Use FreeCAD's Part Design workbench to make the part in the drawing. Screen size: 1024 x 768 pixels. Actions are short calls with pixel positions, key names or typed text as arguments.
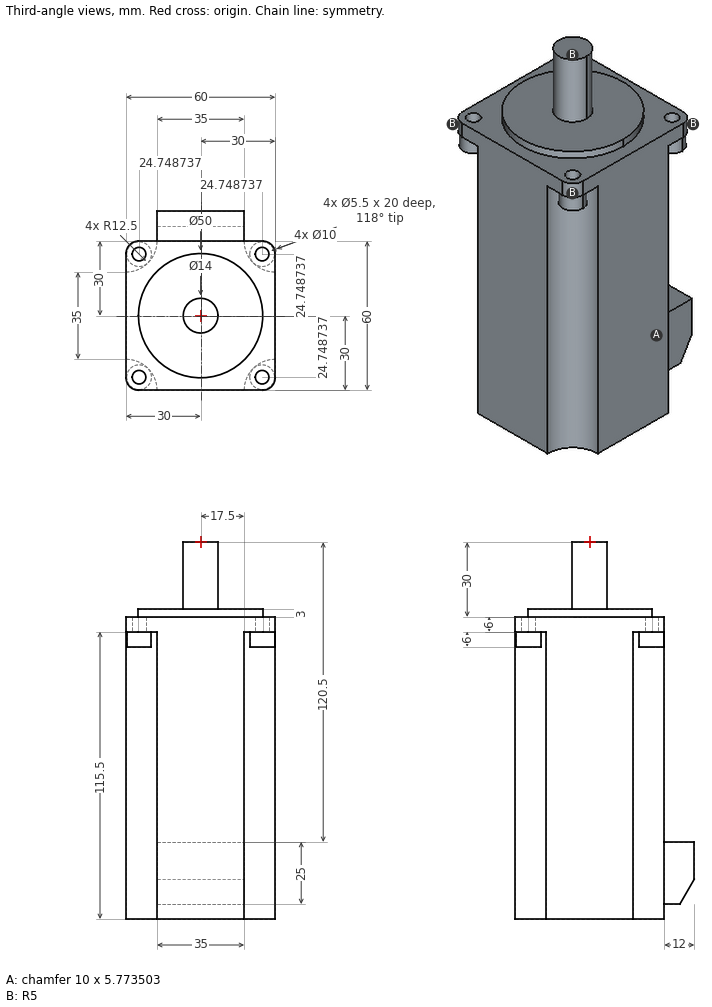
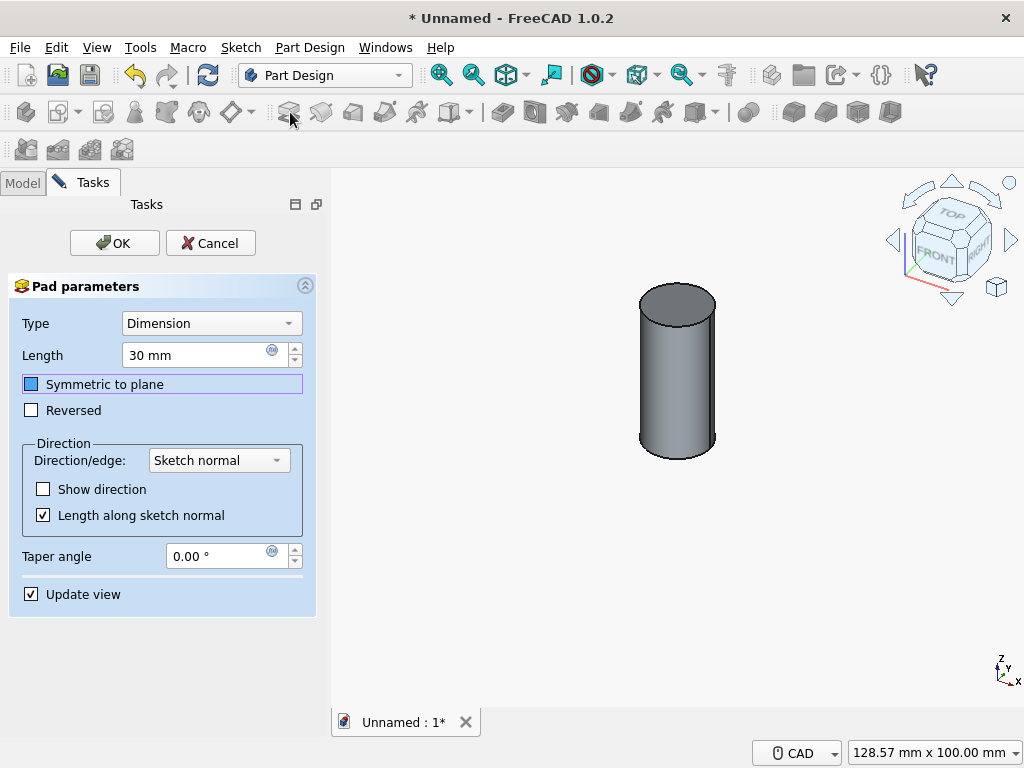
click(30, 410)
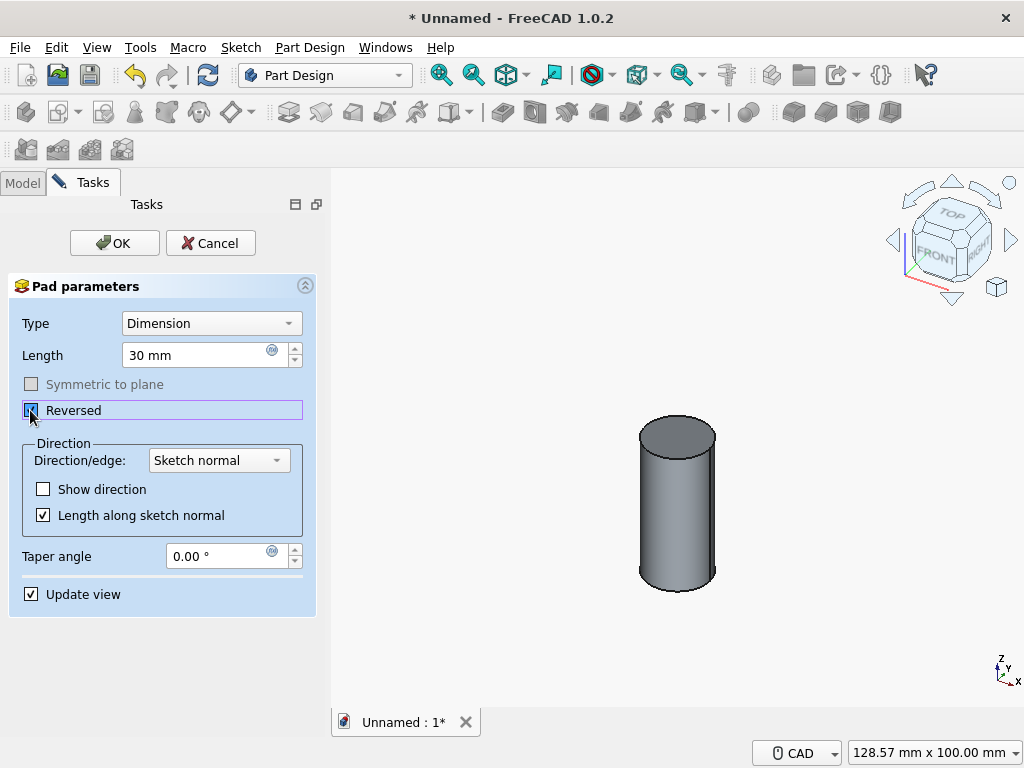
click(115, 243)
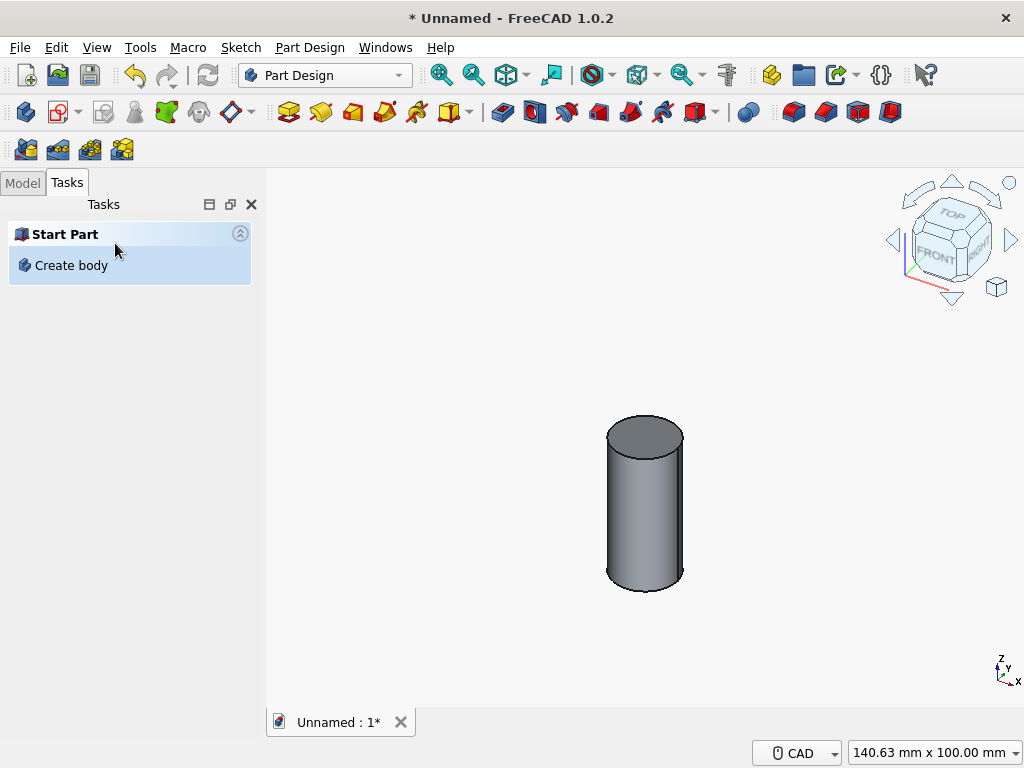
click(442, 76)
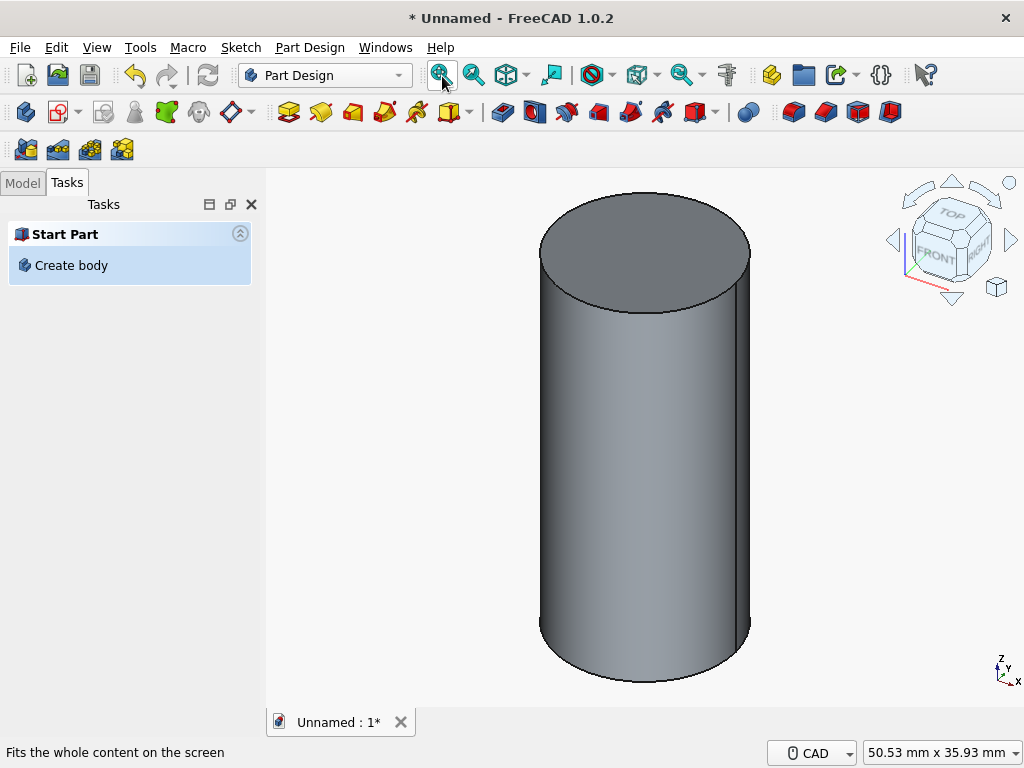
key(5)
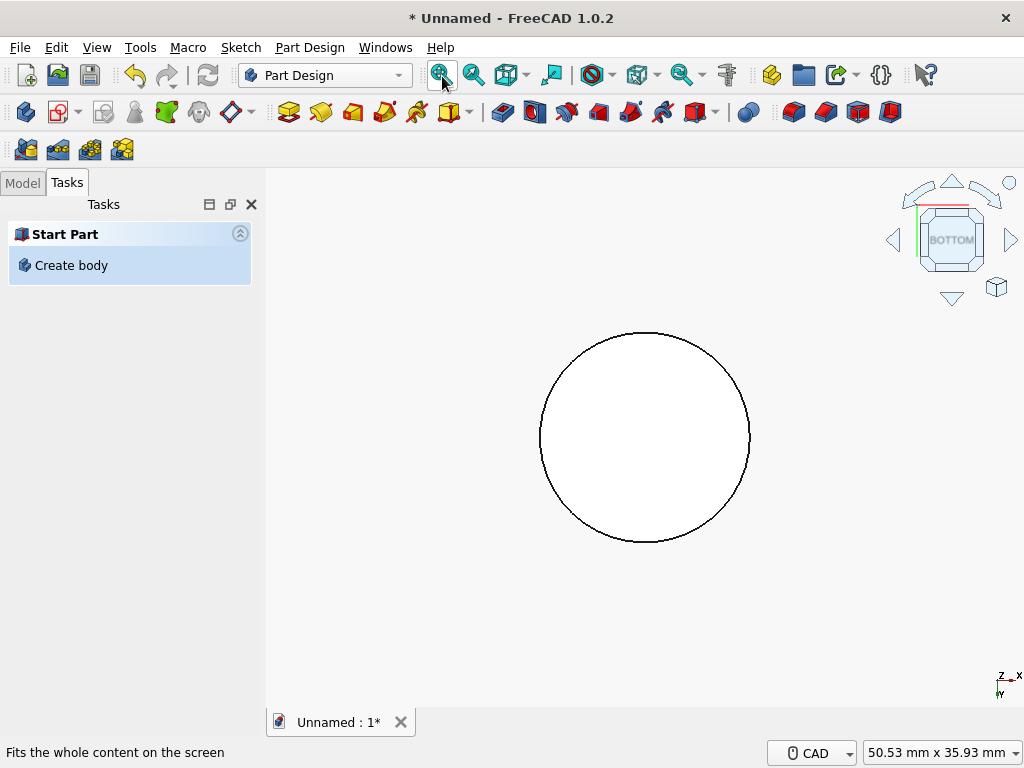
click(442, 76)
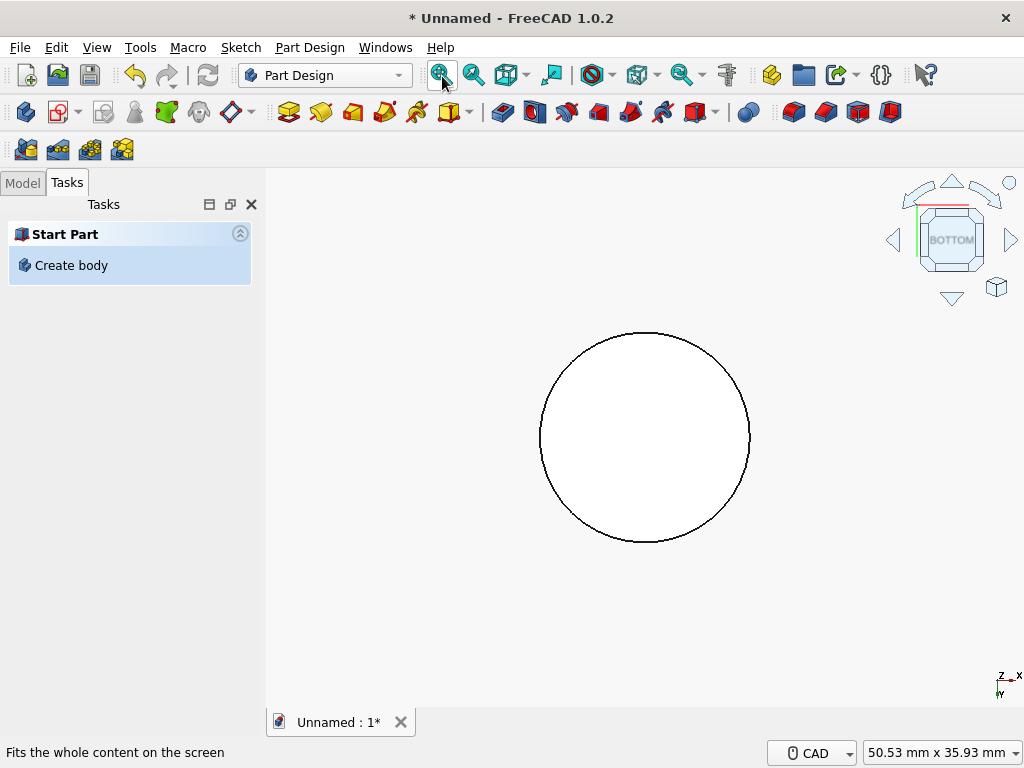
click(645, 436)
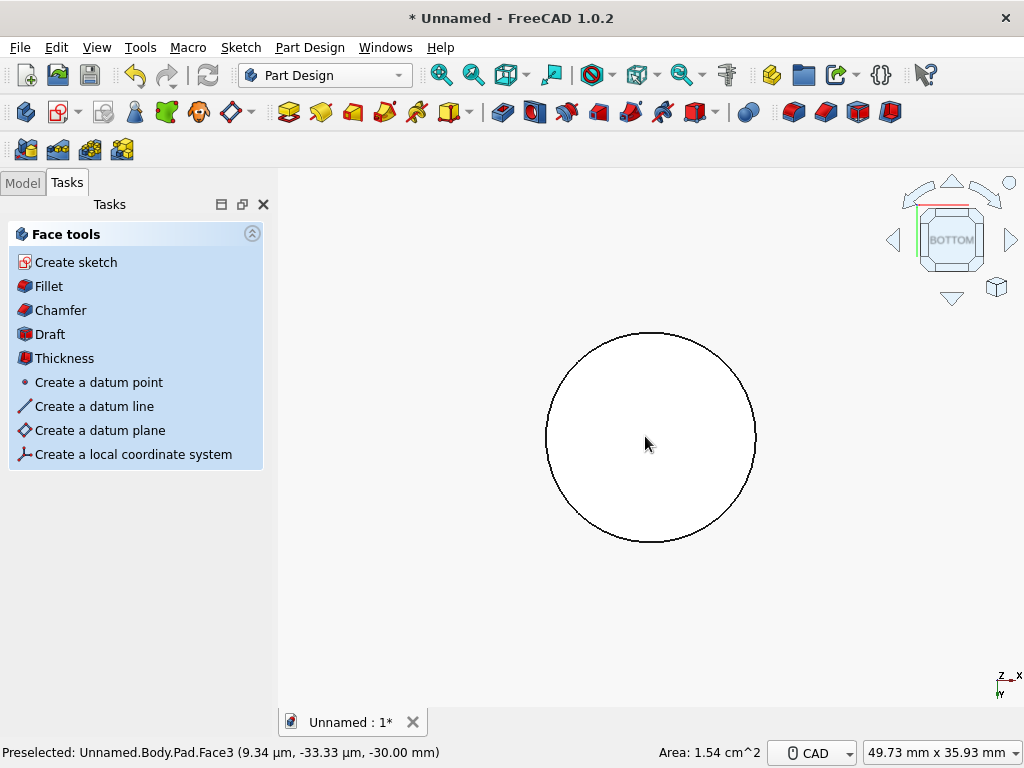
click(58, 112)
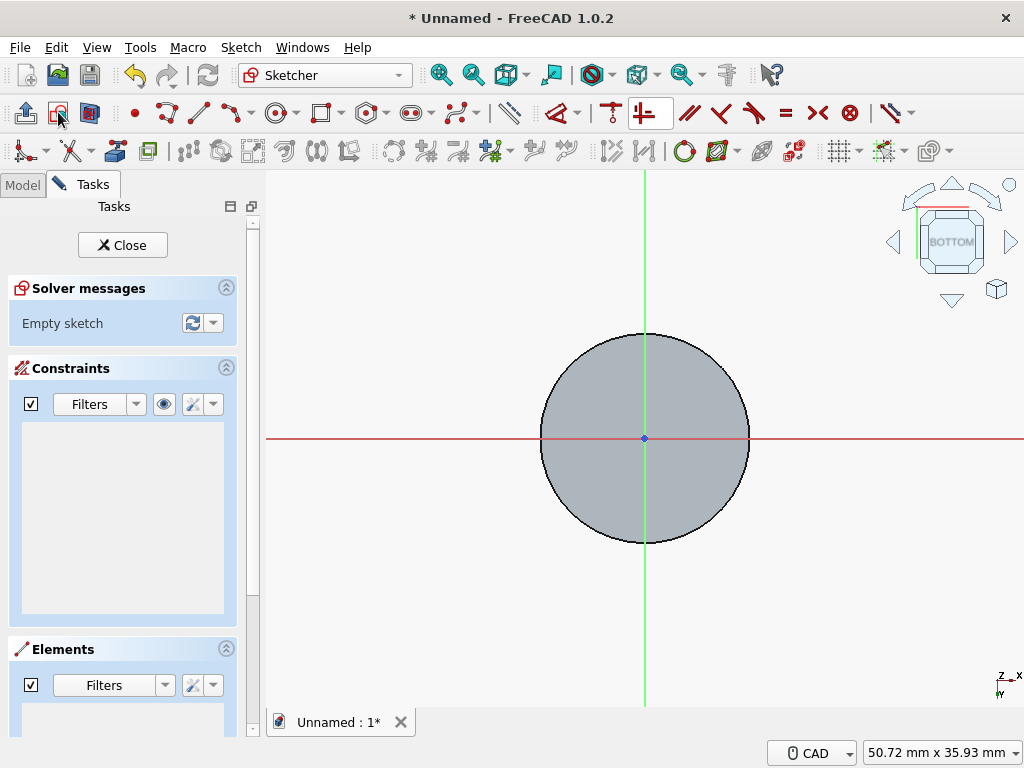
scroll(521, 438, down, 4)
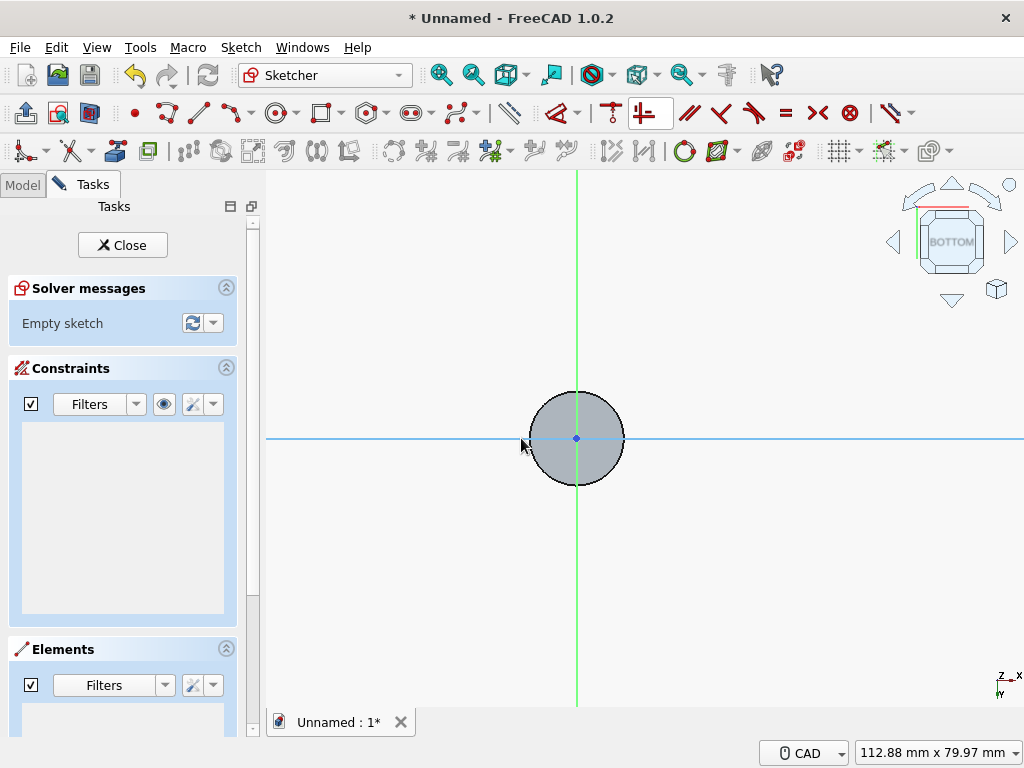
click(276, 114)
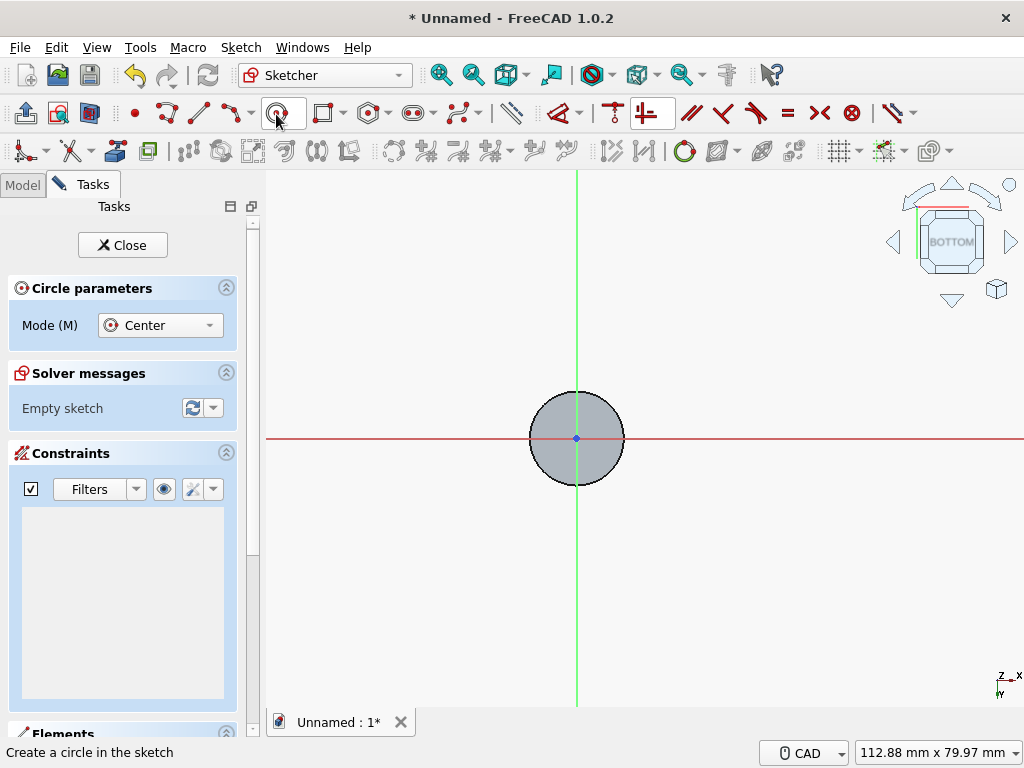
click(577, 438)
click(696, 320)
key(Escape)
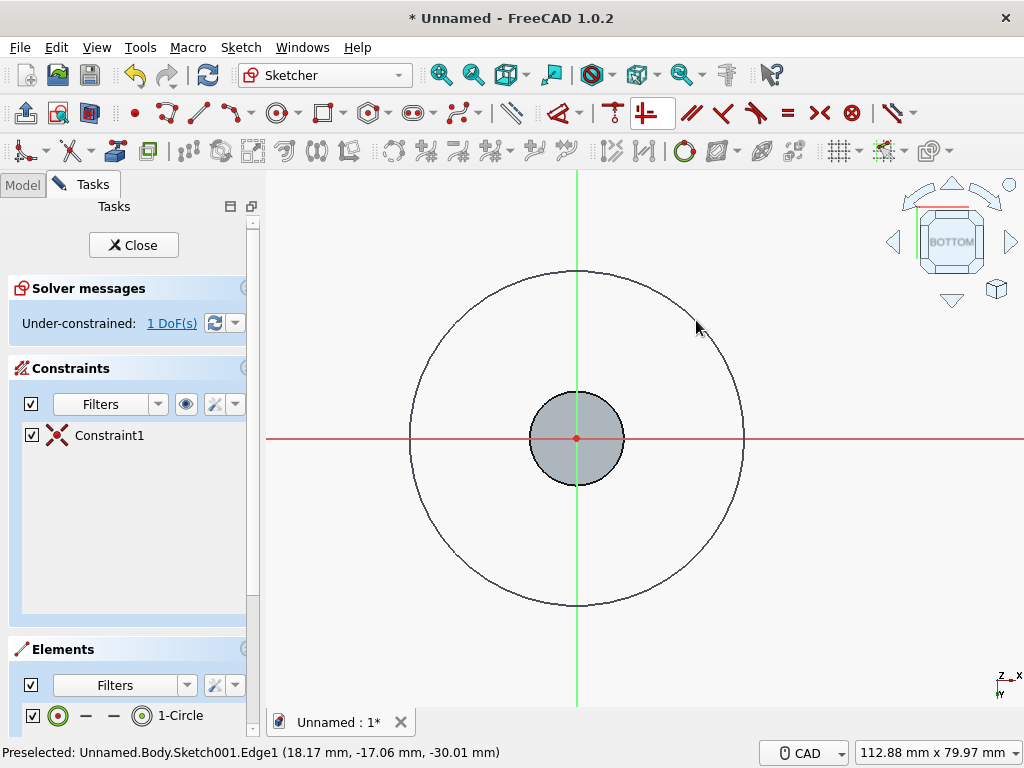
click(558, 114)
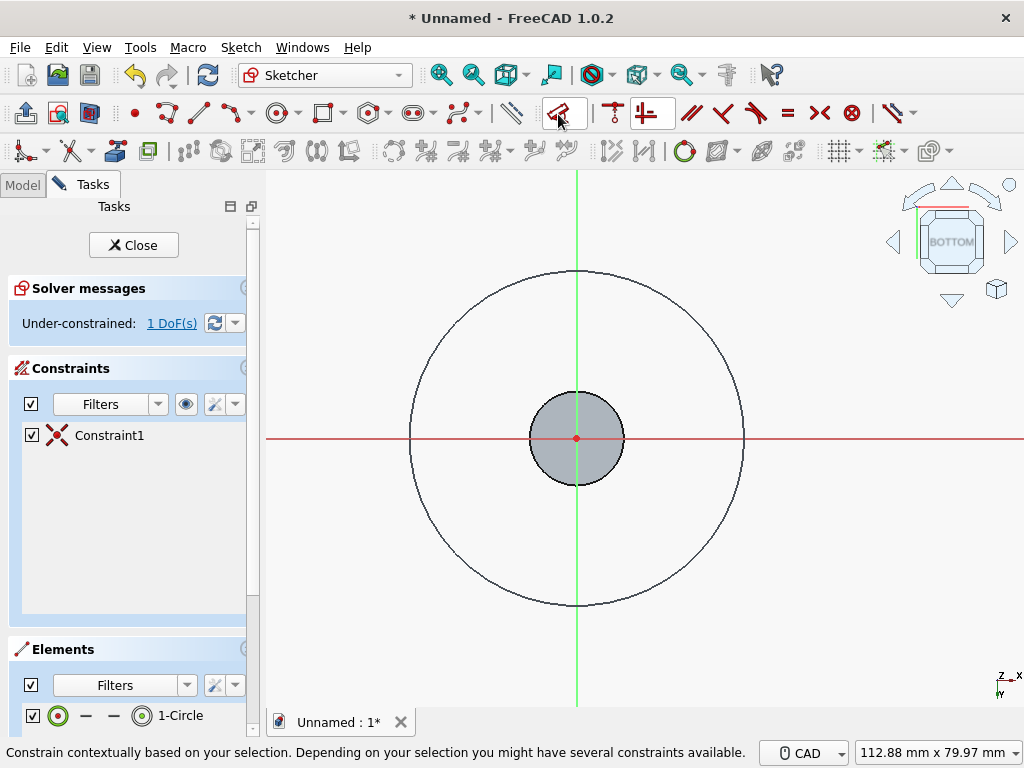
click(695, 320)
click(718, 297)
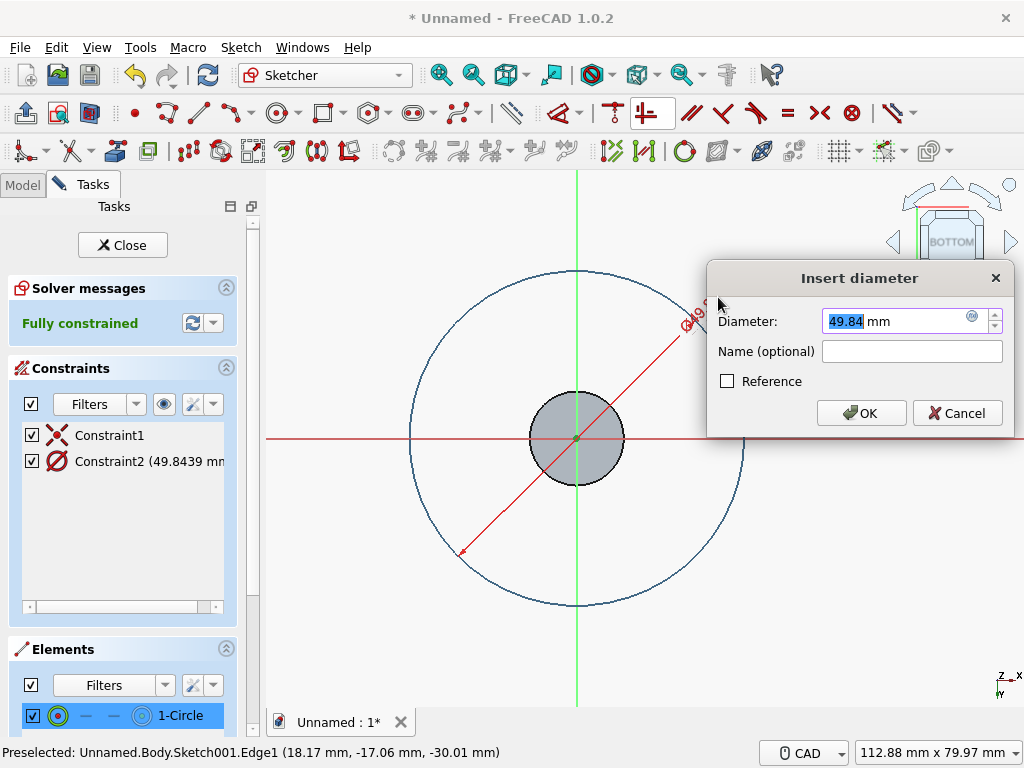
text(50)
key(Return)
key(Escape)